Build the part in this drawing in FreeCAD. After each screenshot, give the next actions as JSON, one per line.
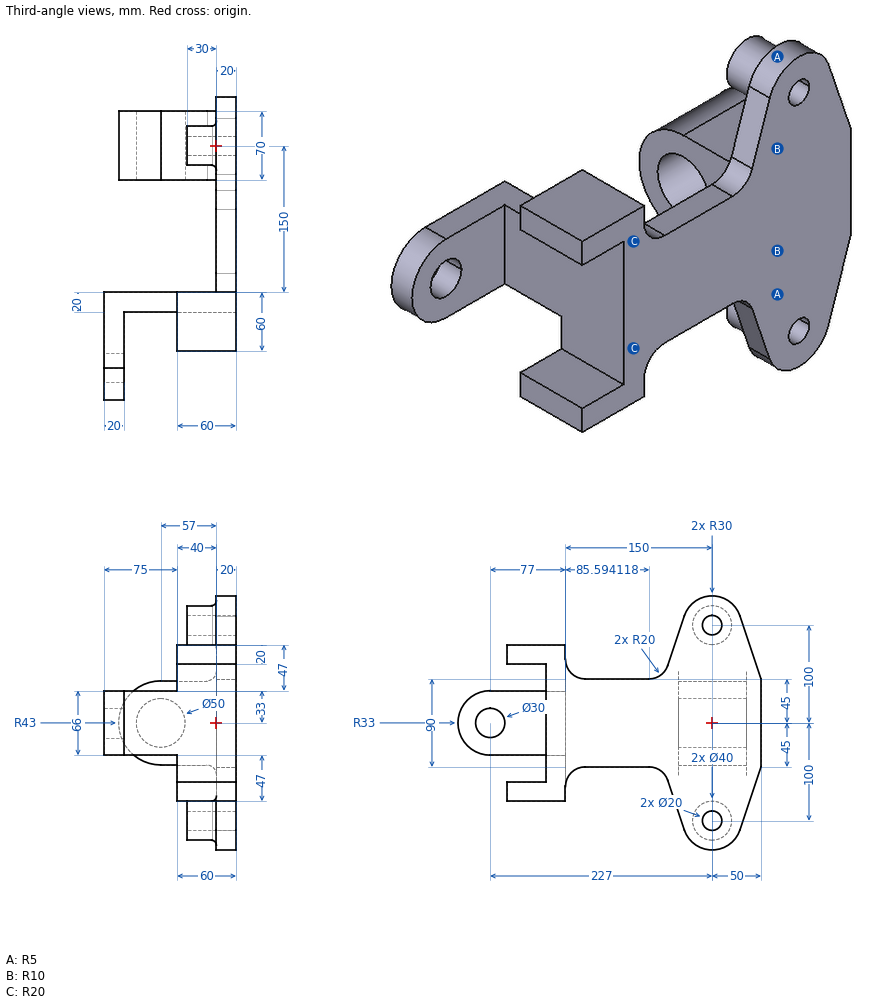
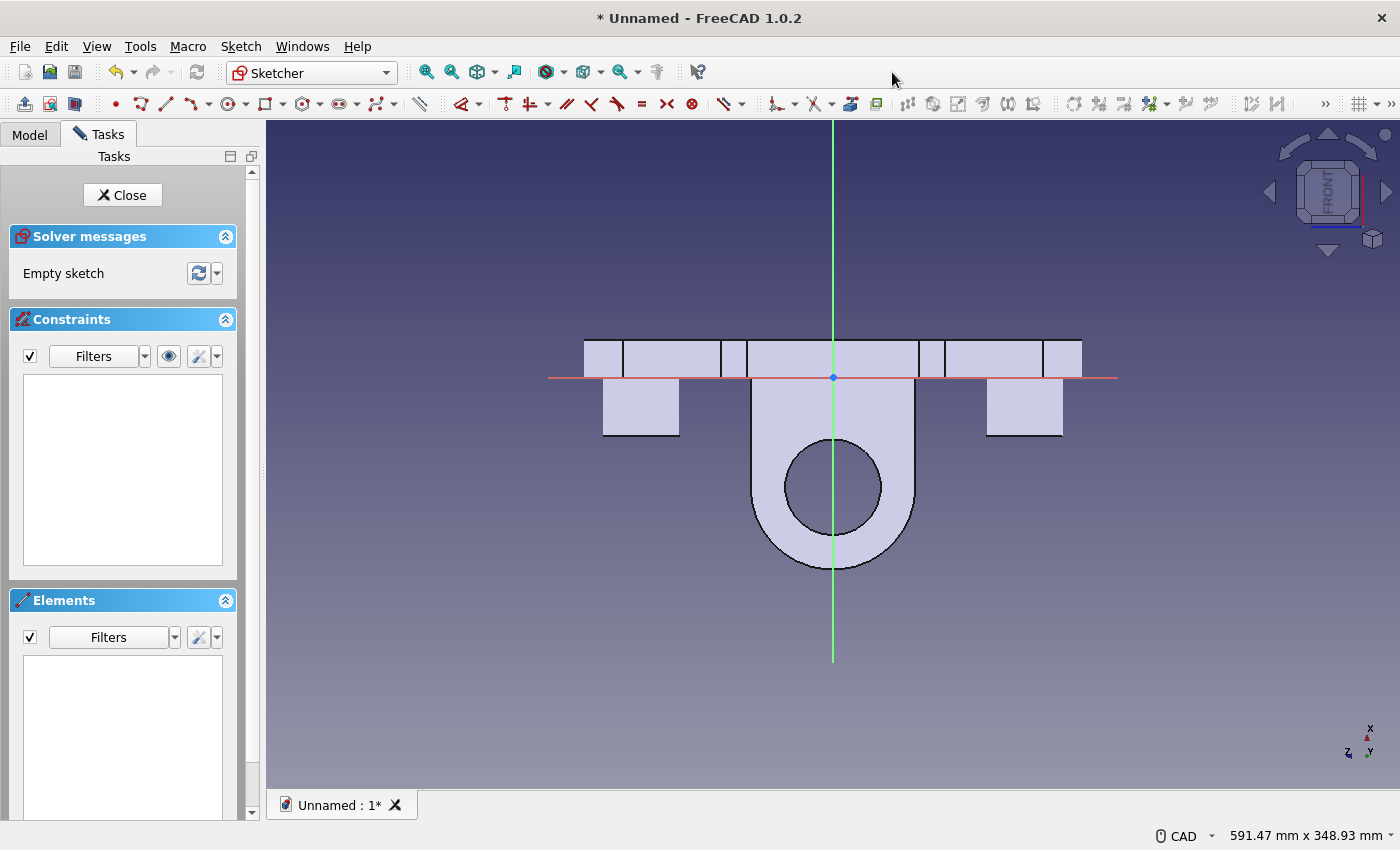
{"action": "scroll", "coordinate": [916, 487], "scroll_direction": "up", "scroll_amount": 3}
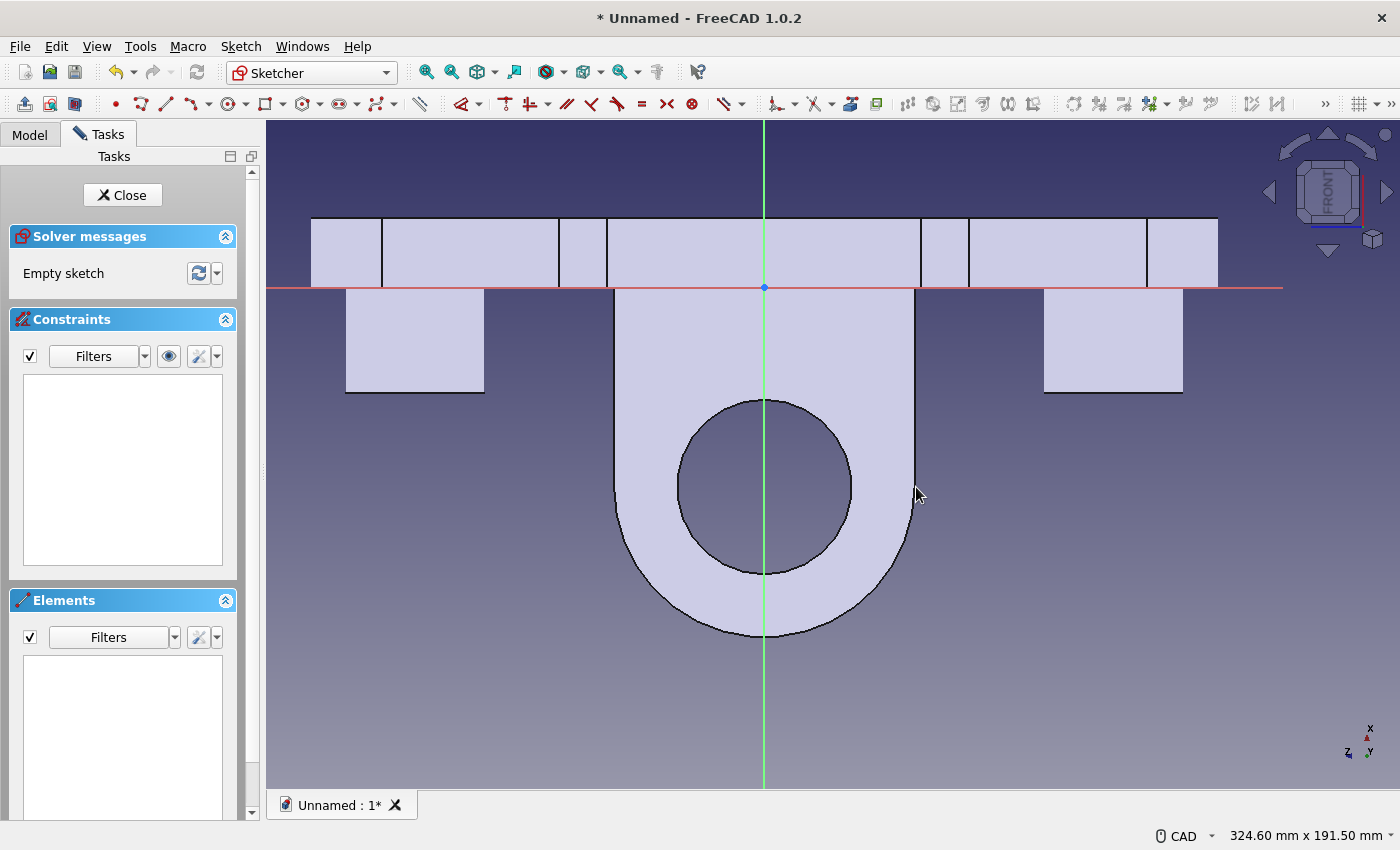
{"action": "key", "text": "g m"}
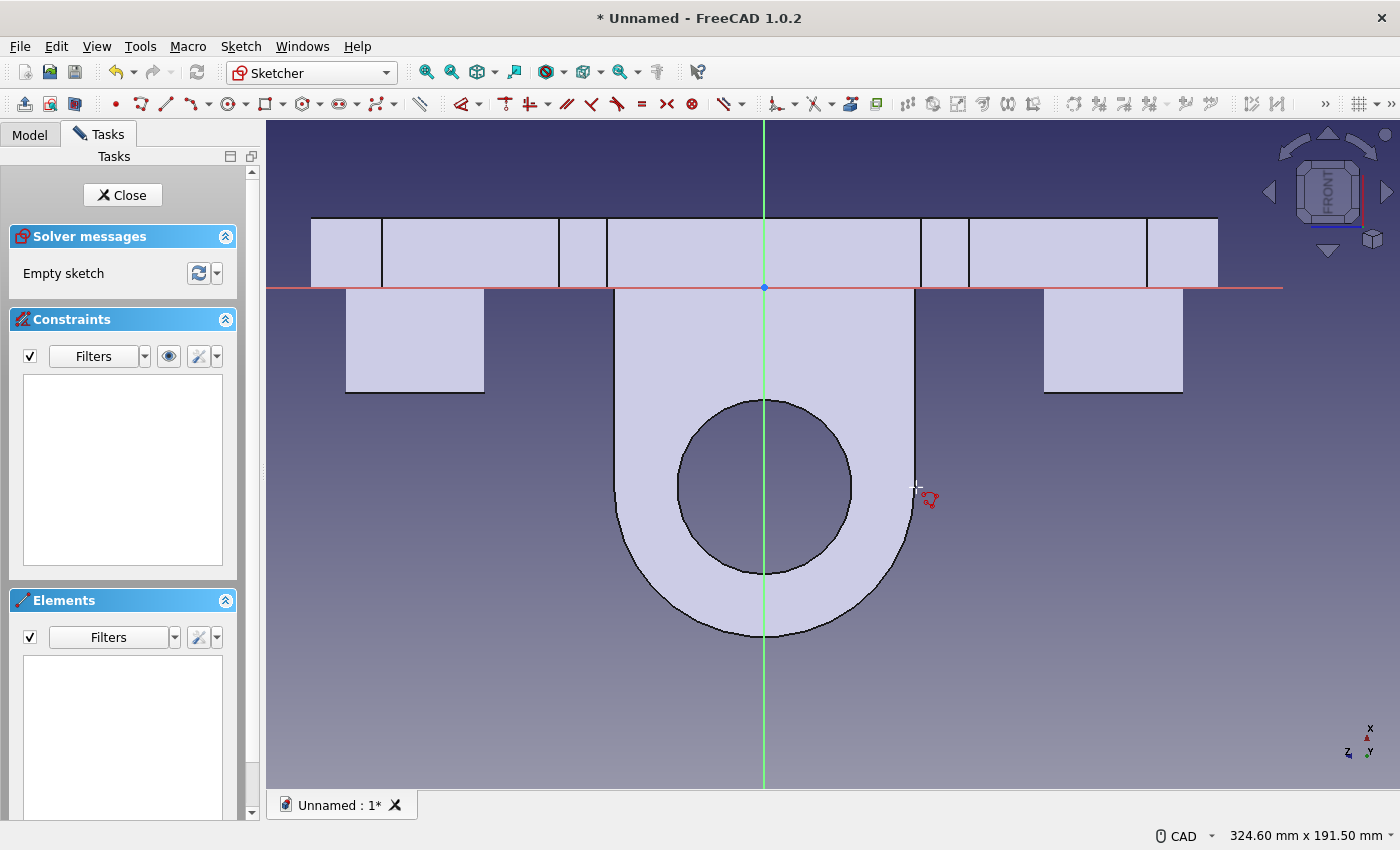
{"action": "left_click", "coordinate": [649, 428]}
{"action": "left_click", "coordinate": [649, 690]}
{"action": "left_click", "coordinate": [880, 690]}
{"action": "left_click", "coordinate": [880, 428]}
{"action": "left_click", "coordinate": [1044, 428]}
{"action": "left_click", "coordinate": [1044, 218]}
{"action": "left_click", "coordinate": [485, 218]}
{"action": "left_click", "coordinate": [485, 428]}
{"action": "left_click", "coordinate": [649, 429]}
{"action": "key", "text": "Escape"}
{"action": "key", "text": "Escape"}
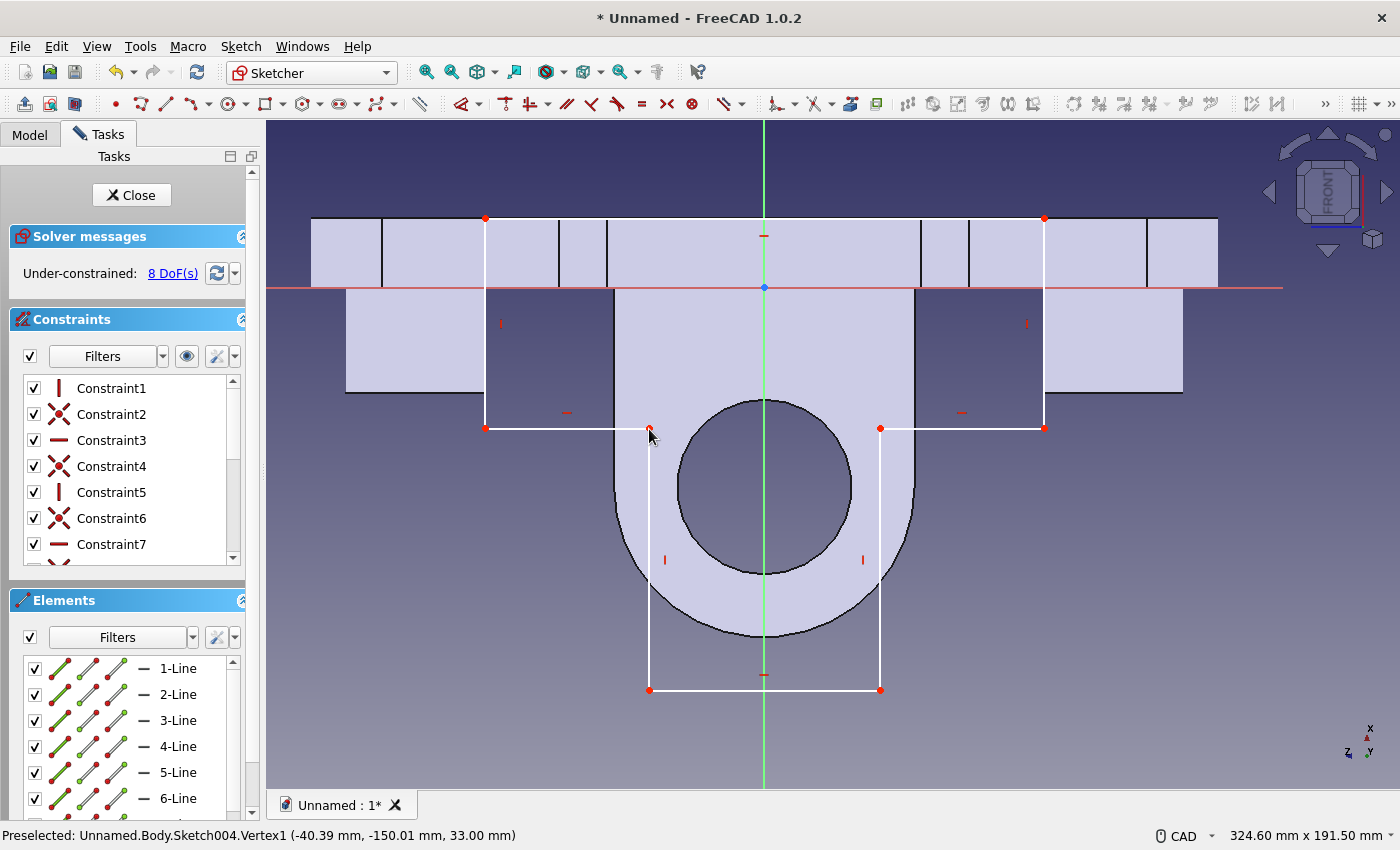
{"action": "key", "text": "d"}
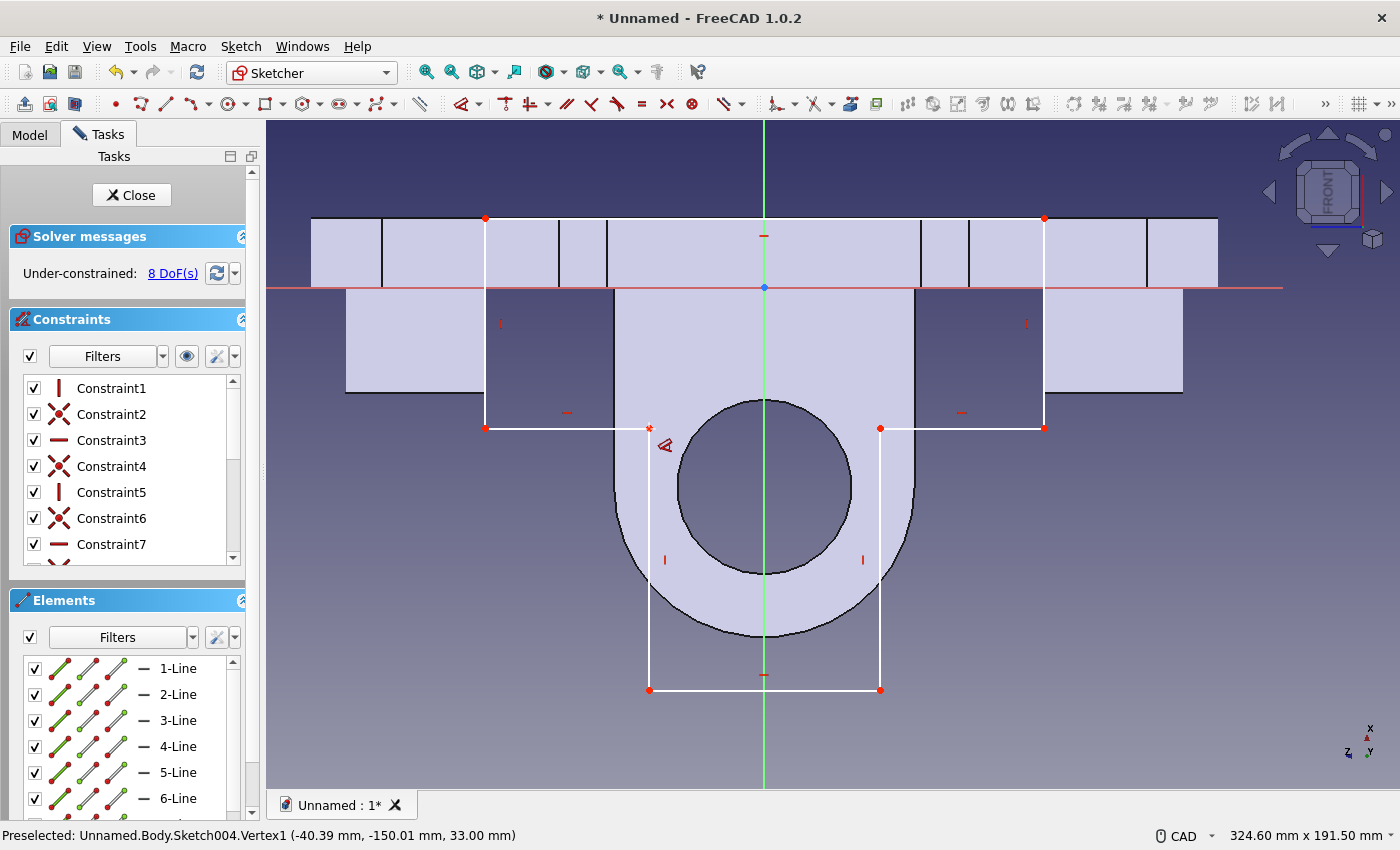
{"action": "left_click", "coordinate": [649, 508]}
{"action": "left_click", "coordinate": [615, 560]}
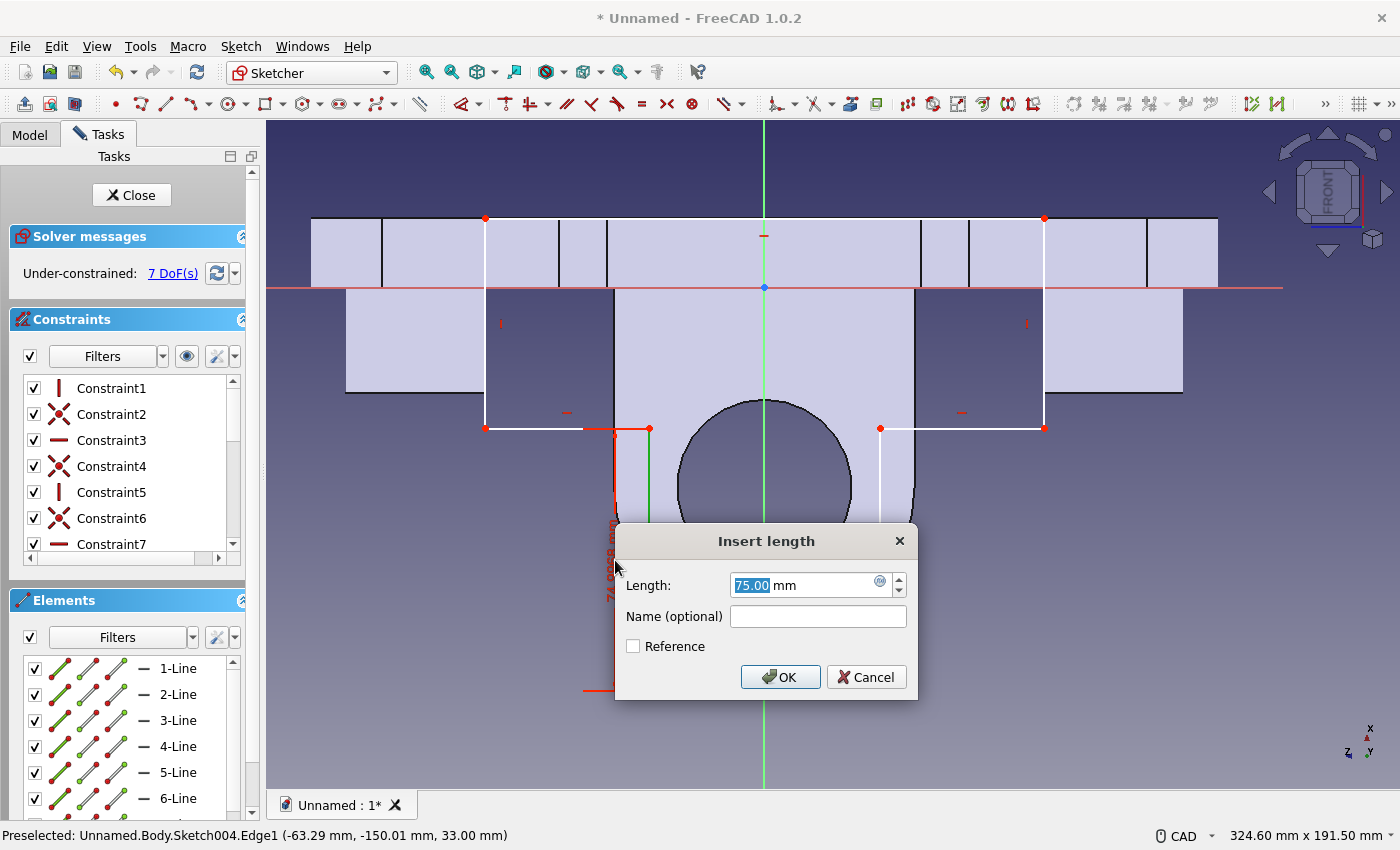
{"action": "type", "text": "75"}
{"action": "key", "text": "Return"}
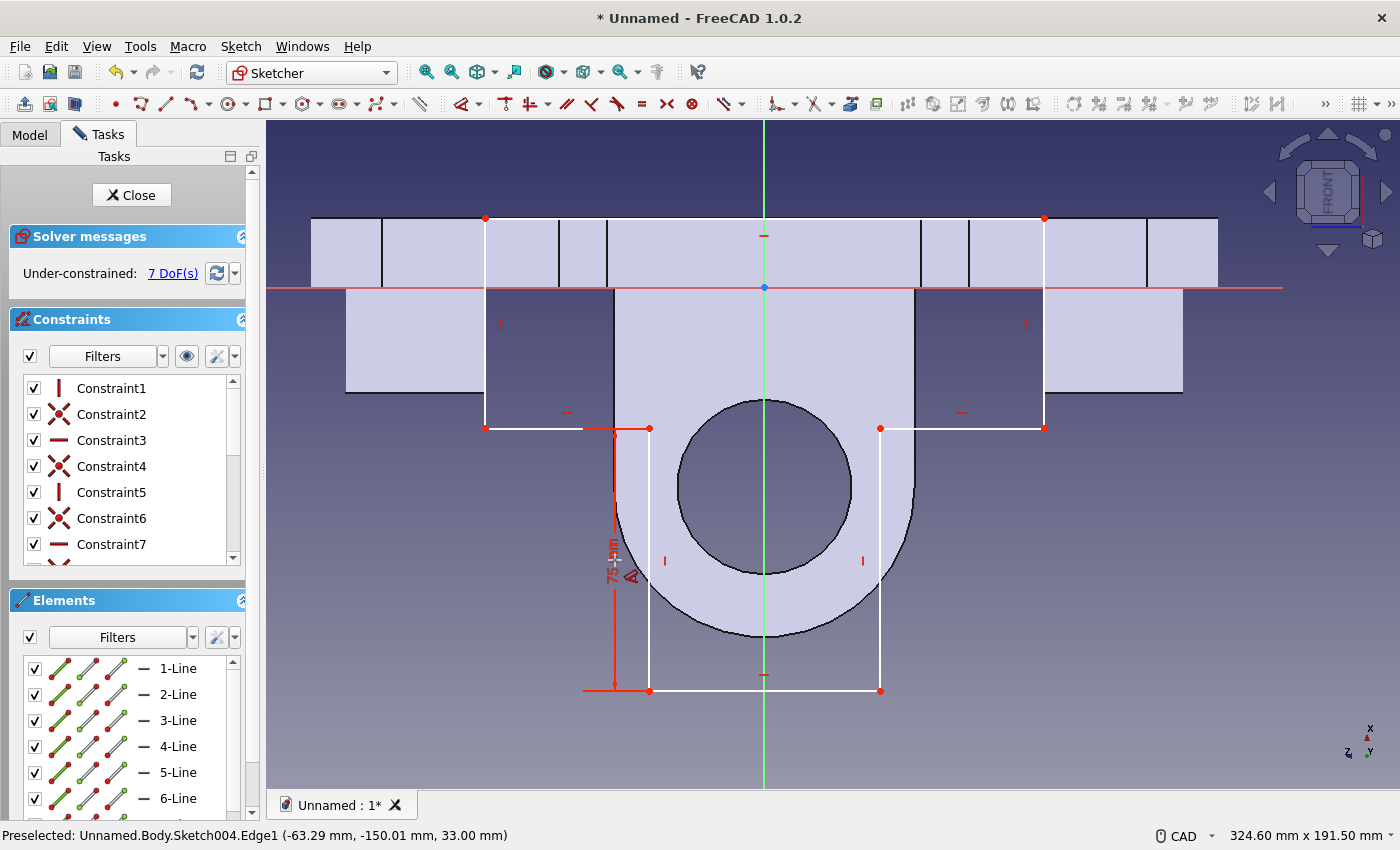
{"action": "left_click", "coordinate": [718, 691]}
{"action": "left_click", "coordinate": [711, 725]}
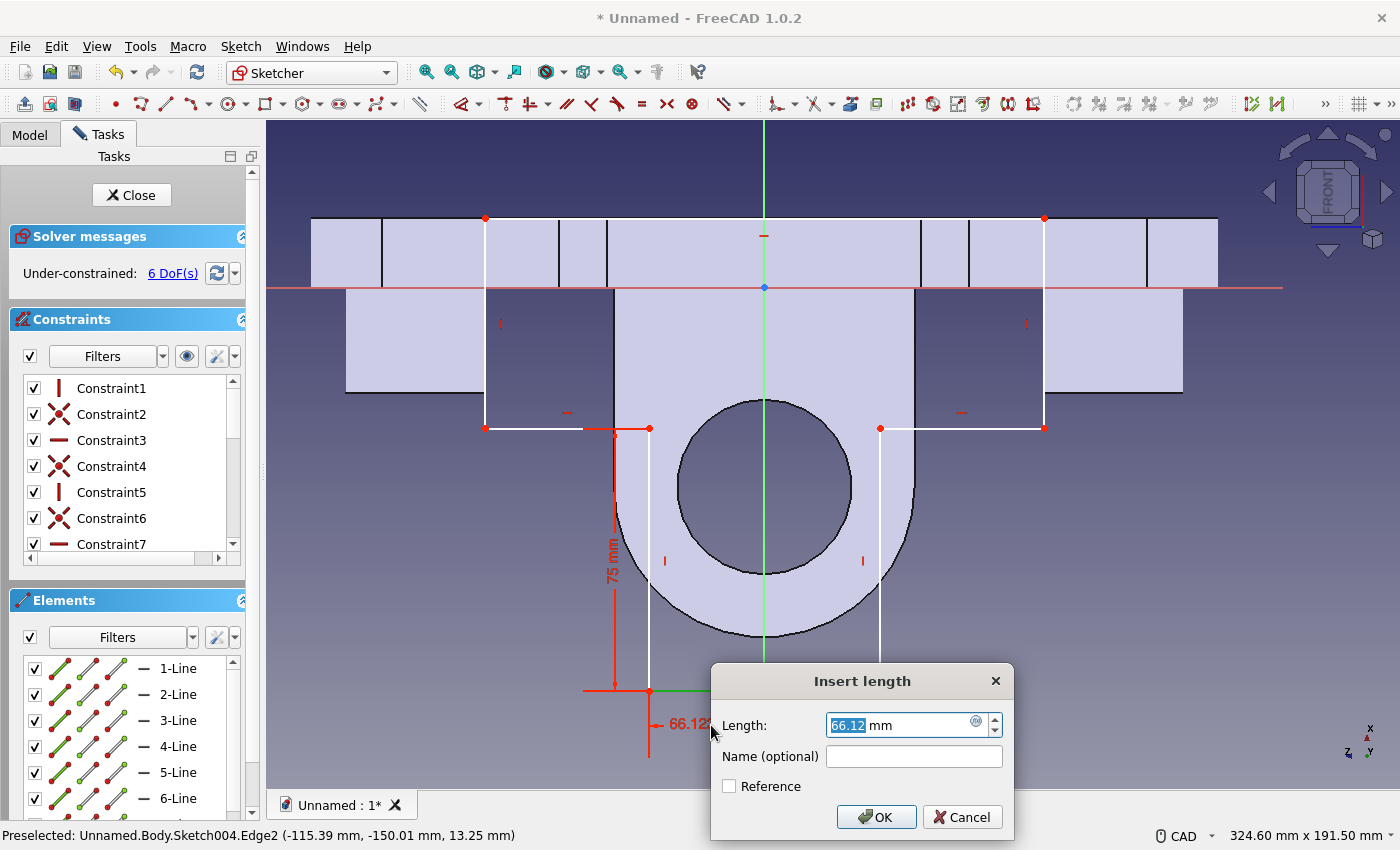
{"action": "type", "text": "66"}
{"action": "key", "text": "Return"}